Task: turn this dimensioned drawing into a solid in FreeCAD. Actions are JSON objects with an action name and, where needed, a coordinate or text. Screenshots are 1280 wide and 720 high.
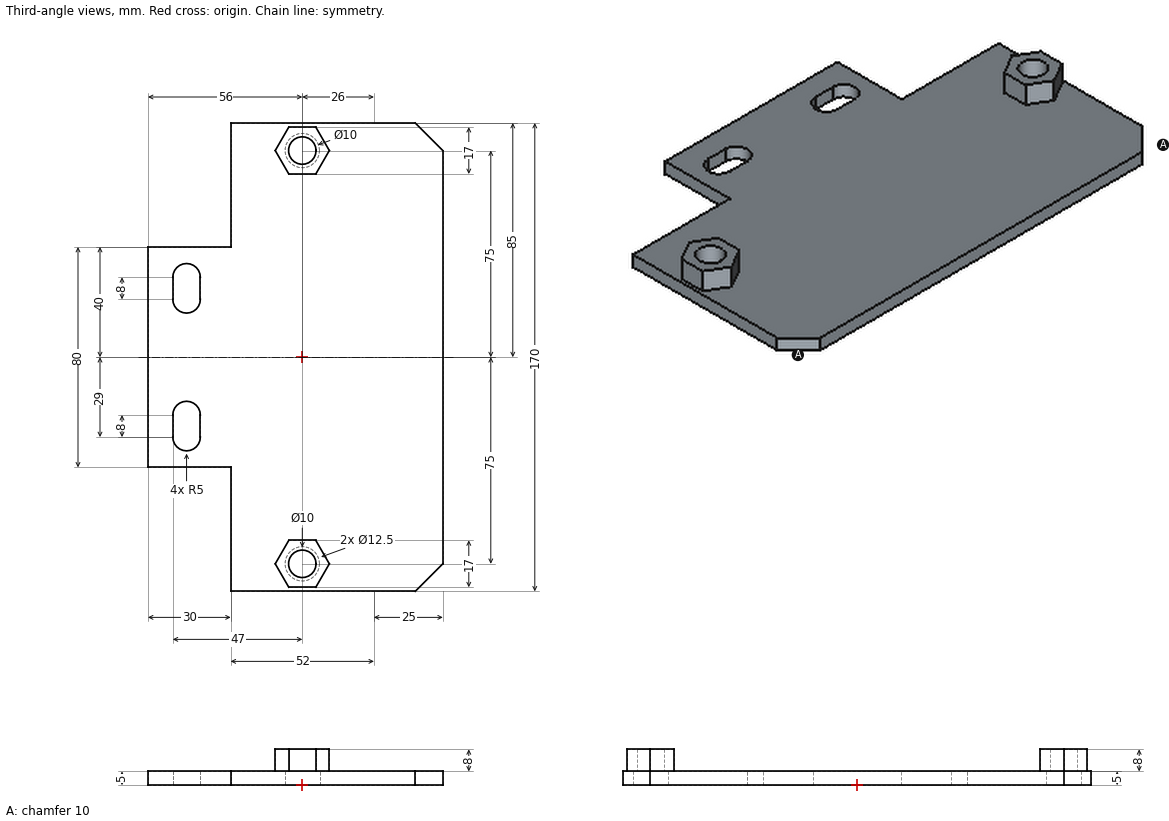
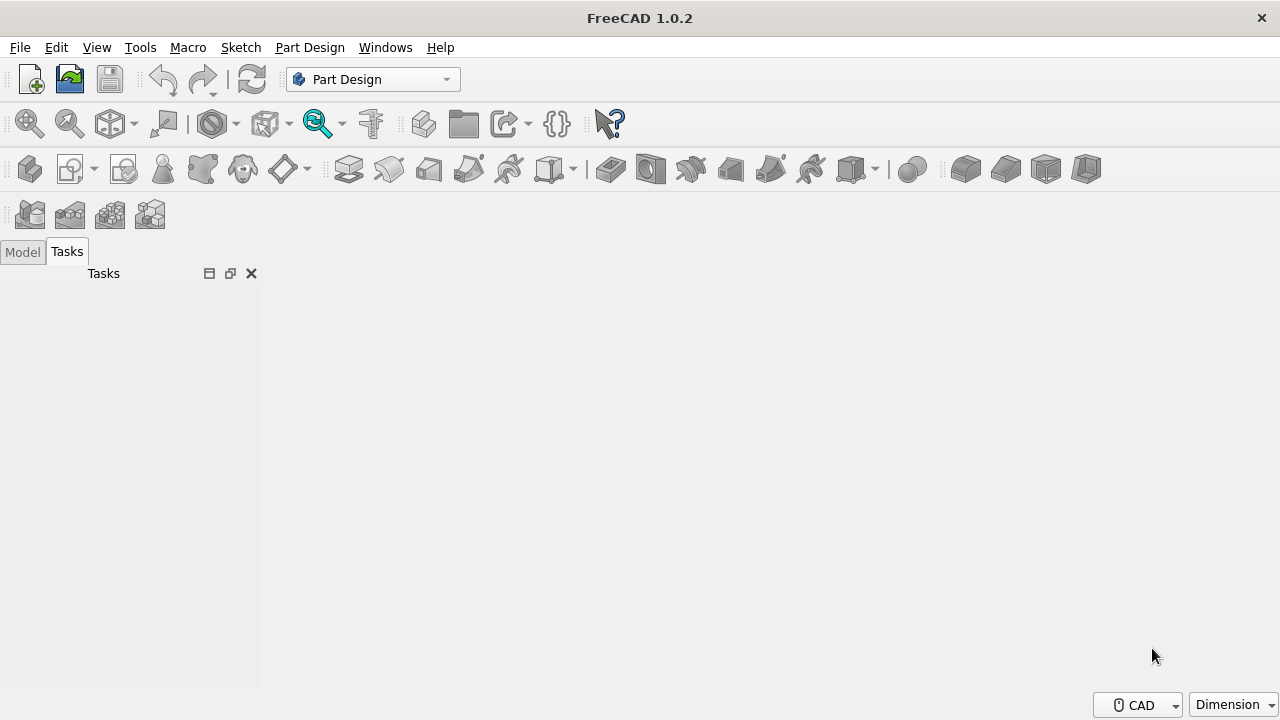
{"action": "left_click", "coordinate": [30, 80]}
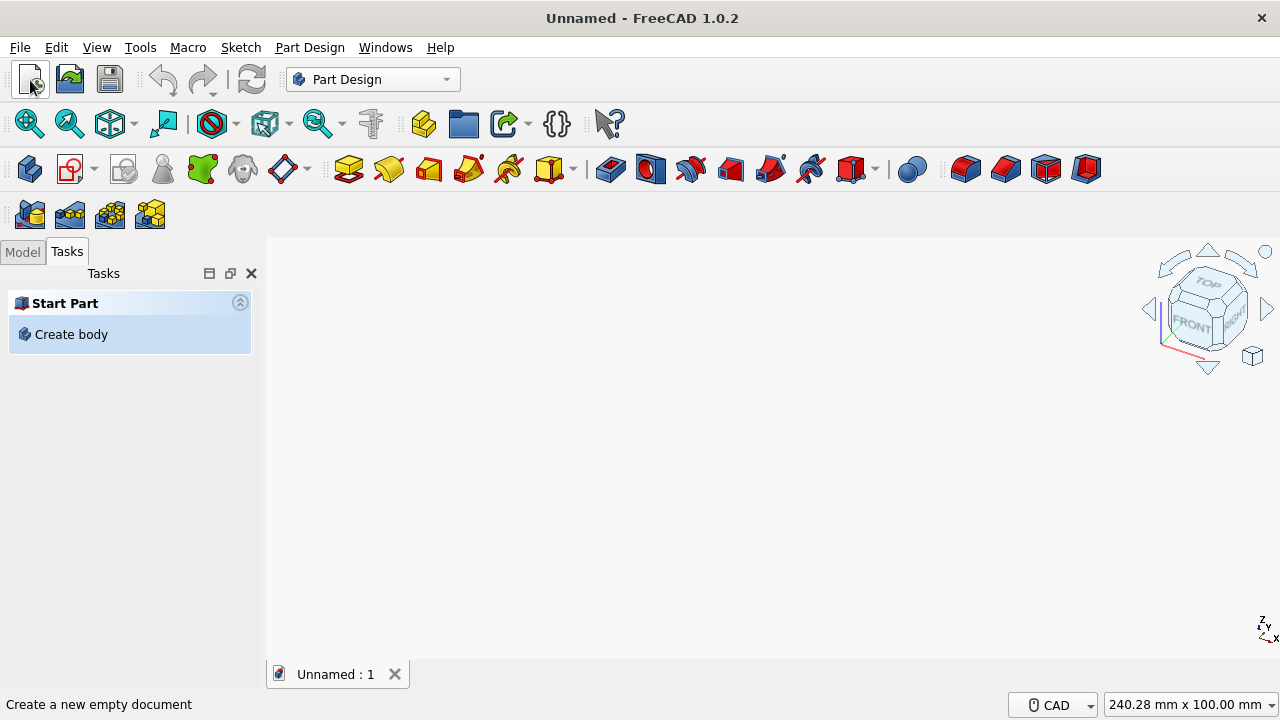
{"action": "left_click", "coordinate": [70, 170]}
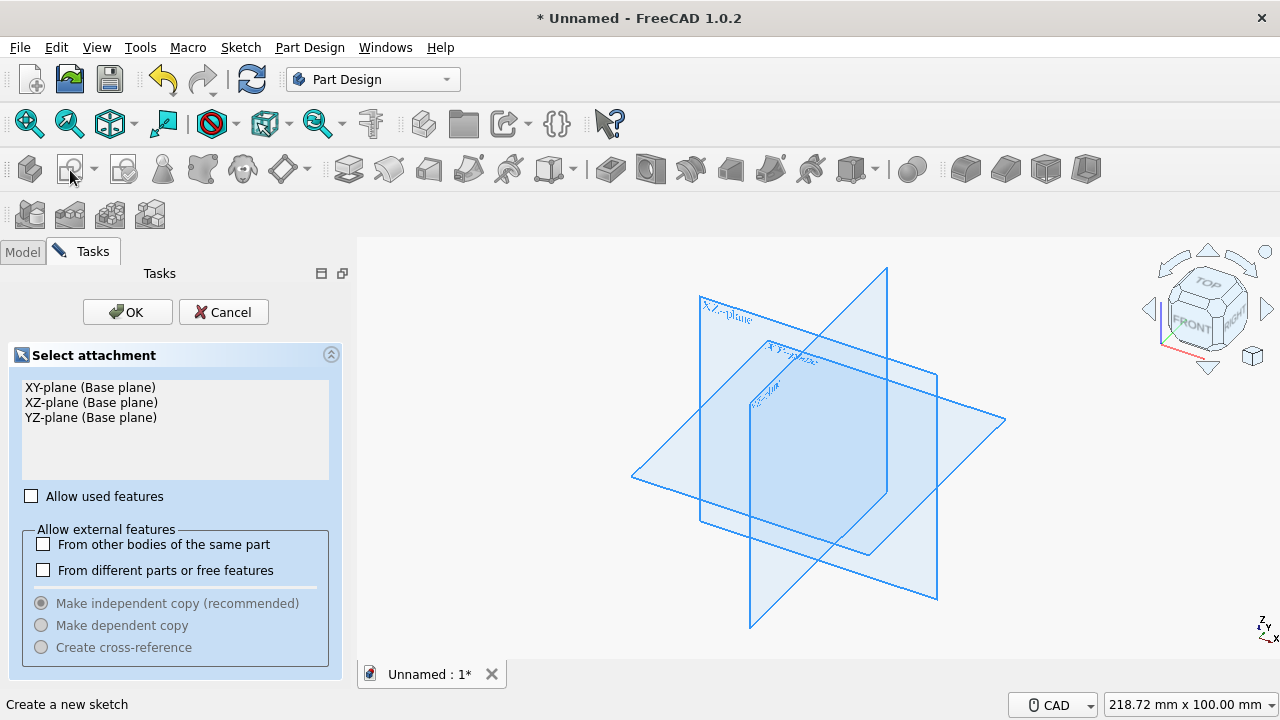
{"action": "left_click", "coordinate": [82, 388]}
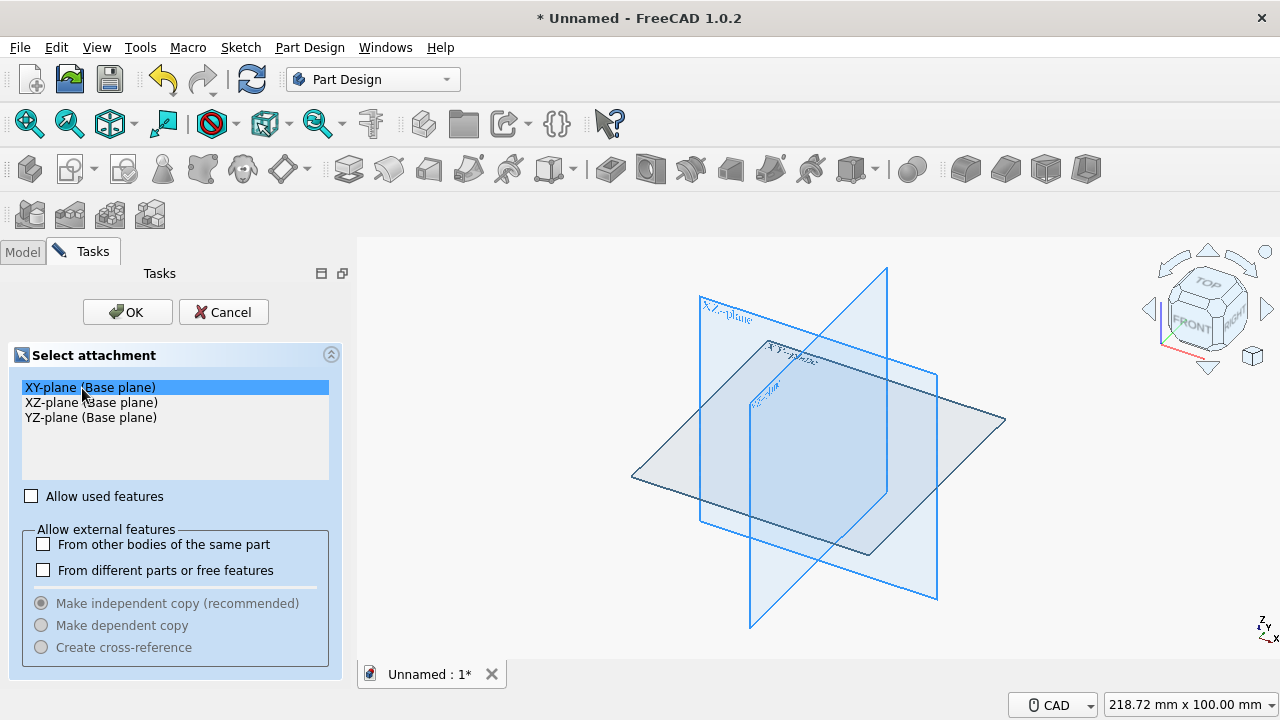
{"action": "left_click", "coordinate": [128, 312]}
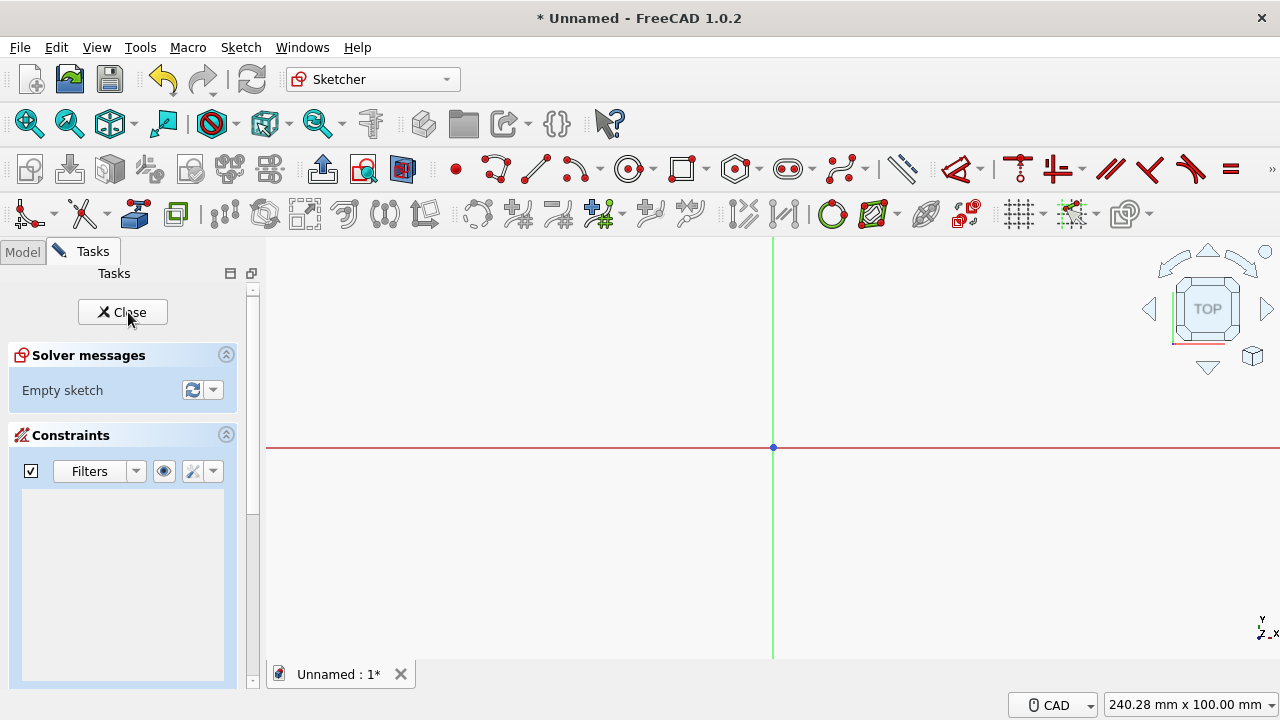
{"action": "scroll", "coordinate": [665, 448], "scroll_direction": "down", "scroll_amount": 5}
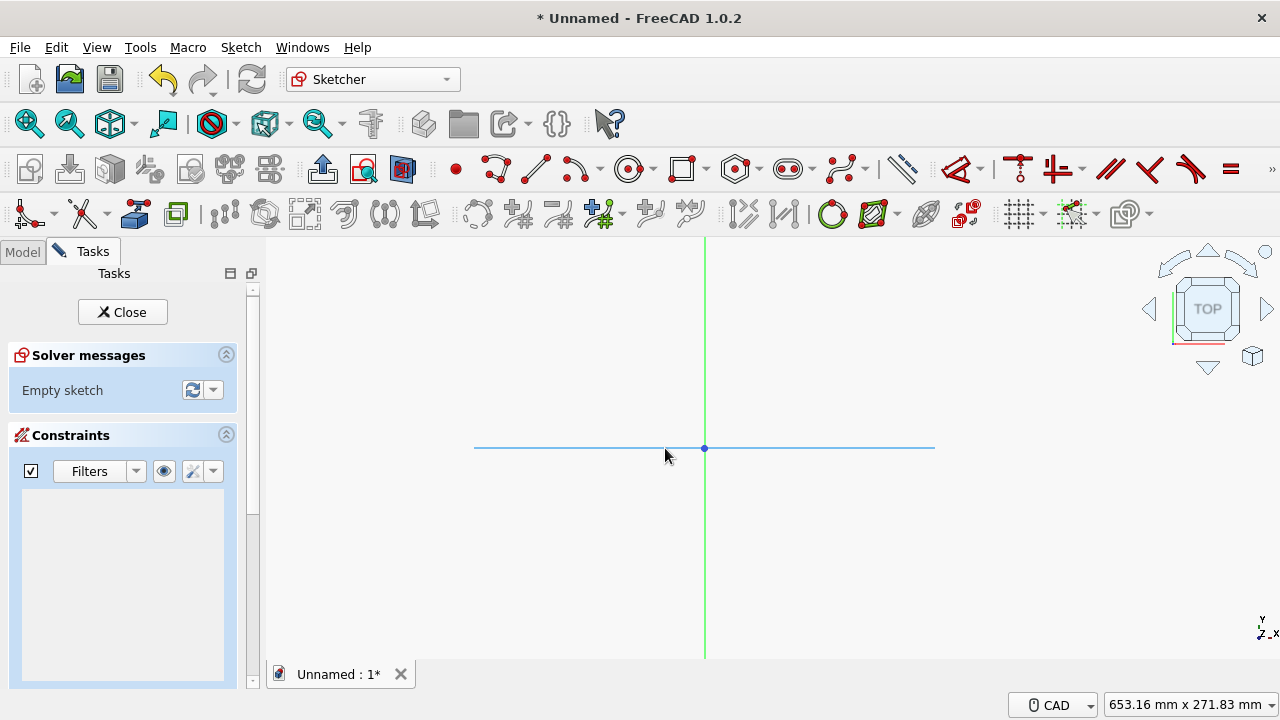
{"action": "key", "text": "g v"}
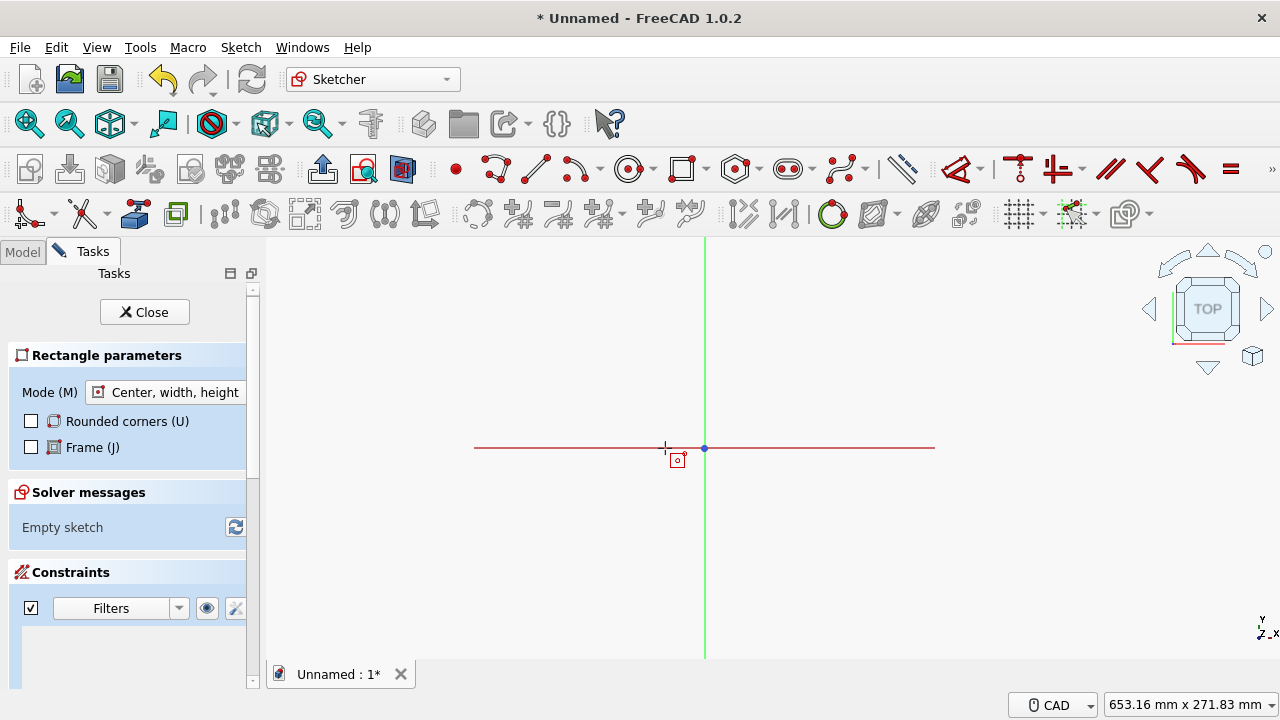
{"action": "left_click", "coordinate": [705, 448]}
{"action": "left_click", "coordinate": [745, 316]}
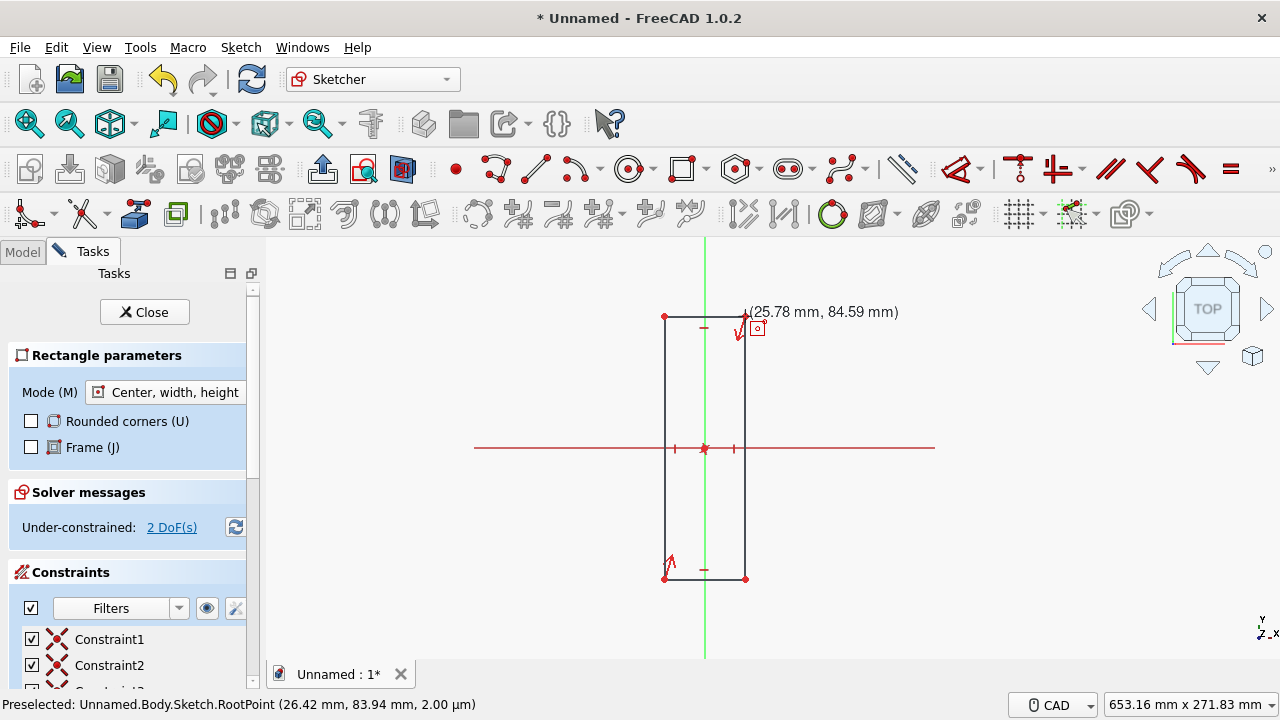
{"action": "left_click", "coordinate": [630, 170]}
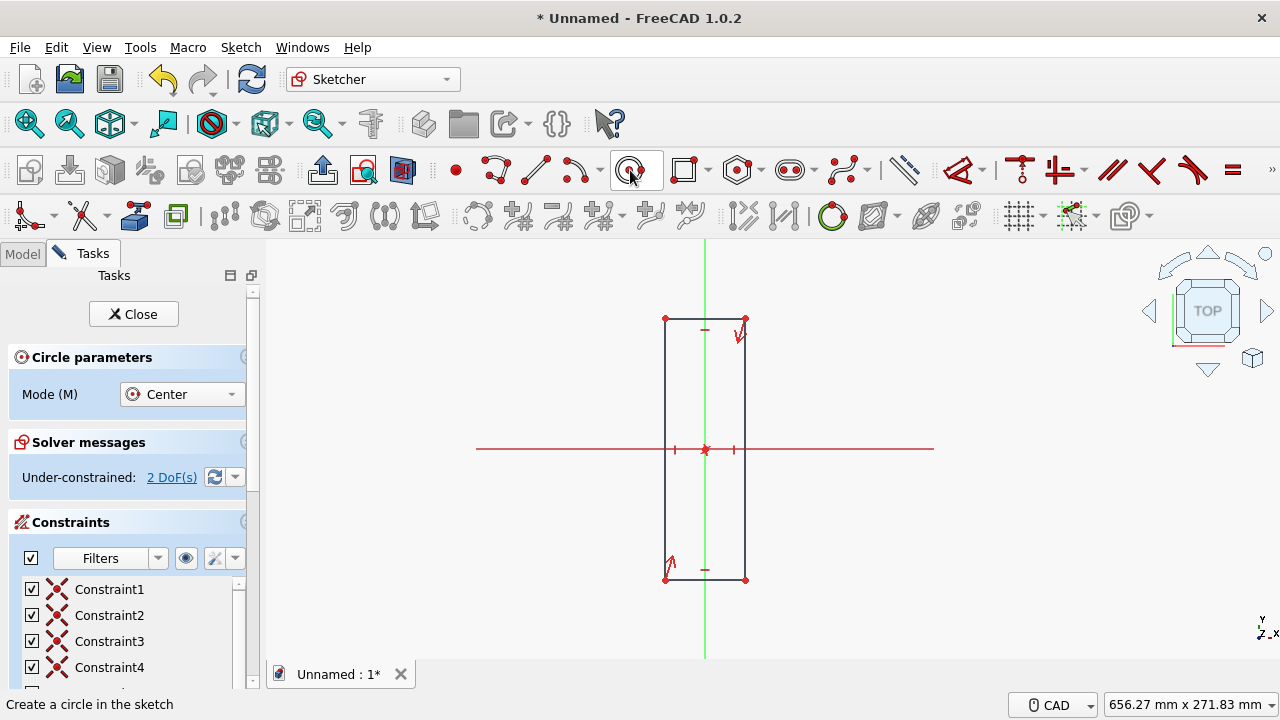
{"action": "scroll", "coordinate": [705, 565], "scroll_direction": "up", "scroll_amount": 5}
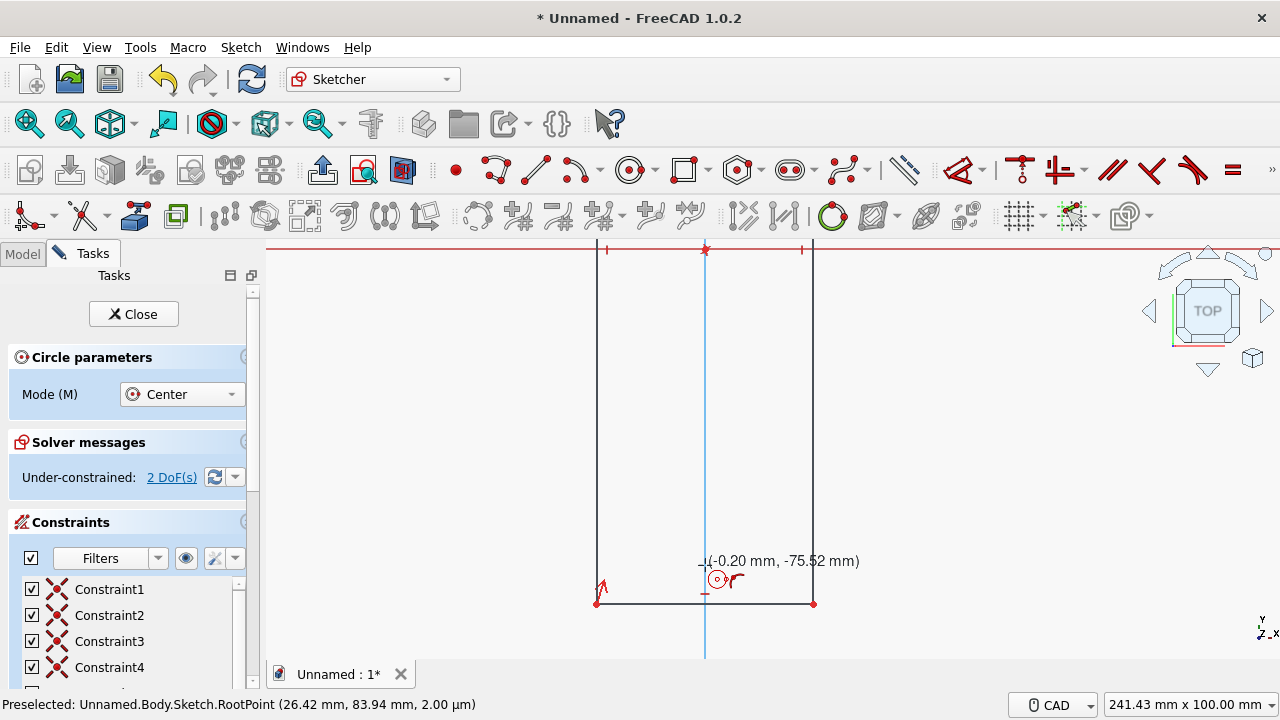
{"action": "left_click", "coordinate": [705, 564]}
{"action": "left_click", "coordinate": [724, 546]}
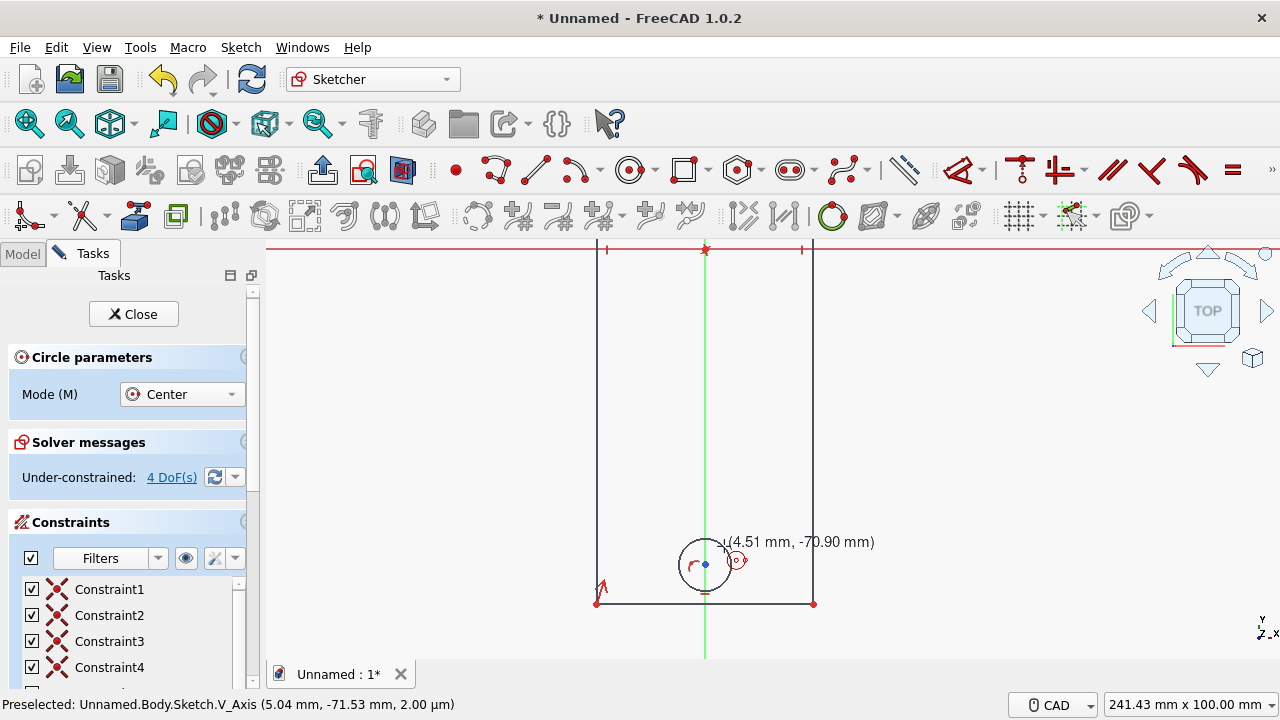
{"action": "scroll", "coordinate": [704, 565], "scroll_direction": "down", "scroll_amount": 5}